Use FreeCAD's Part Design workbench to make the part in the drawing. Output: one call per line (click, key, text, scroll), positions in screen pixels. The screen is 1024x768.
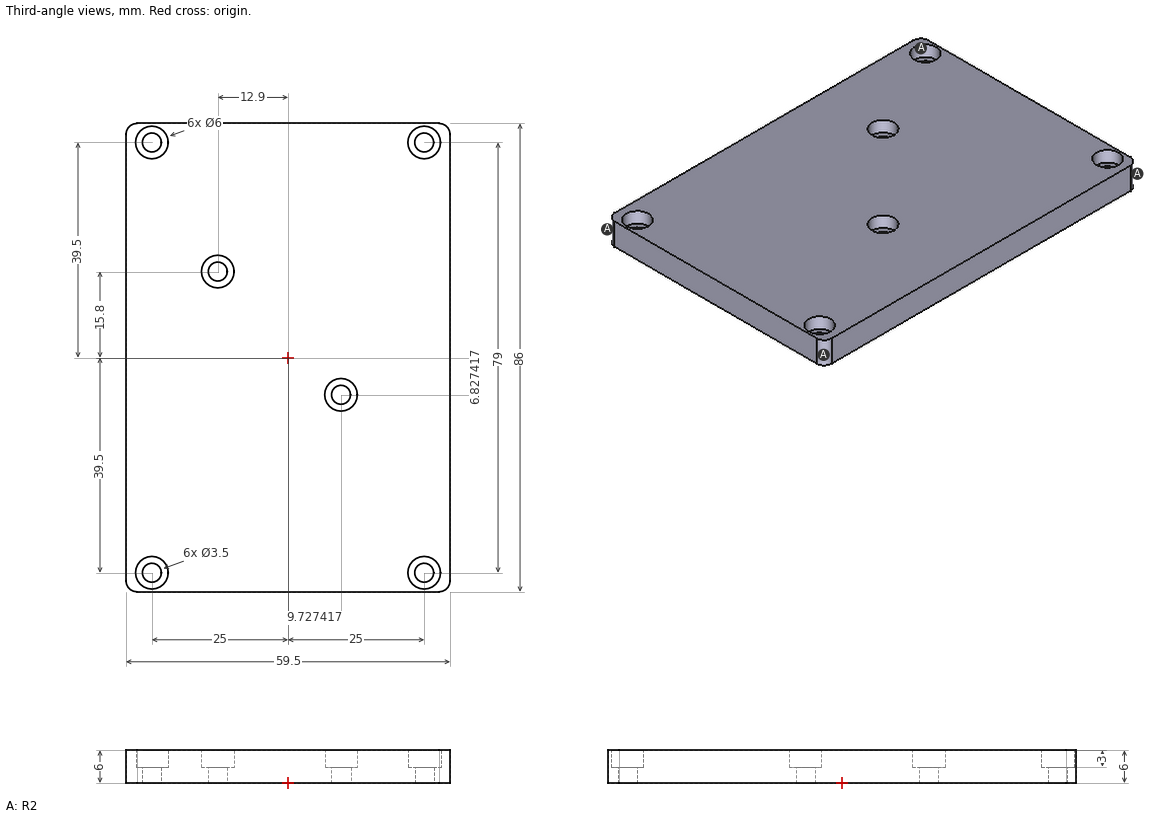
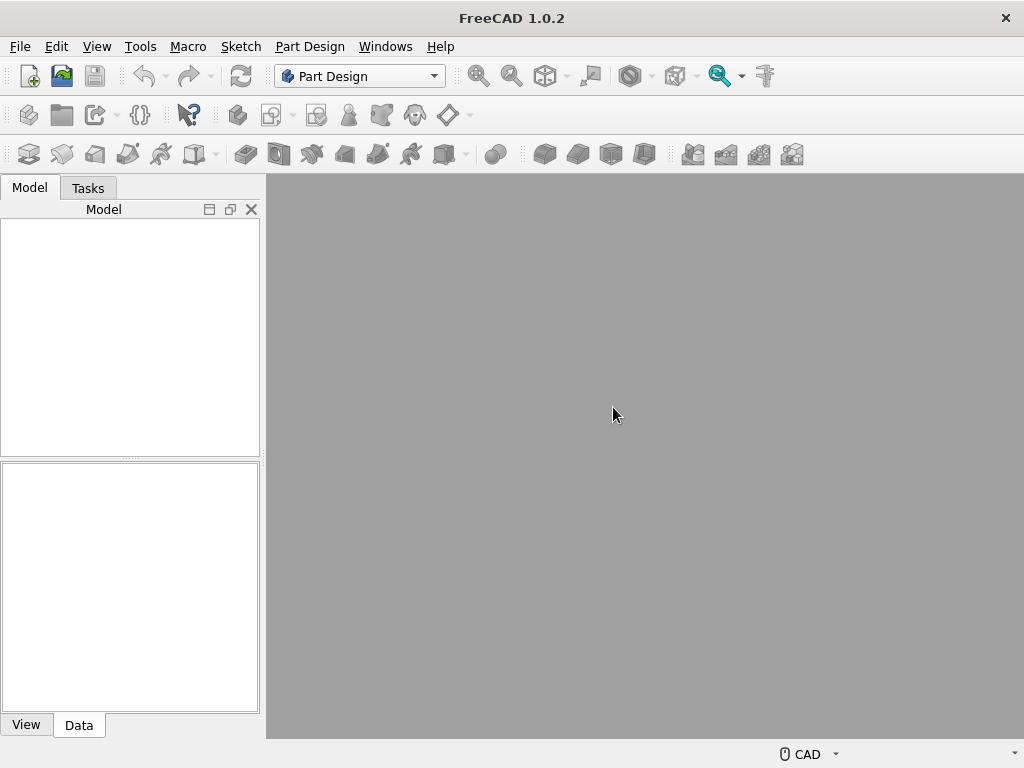
click(29, 76)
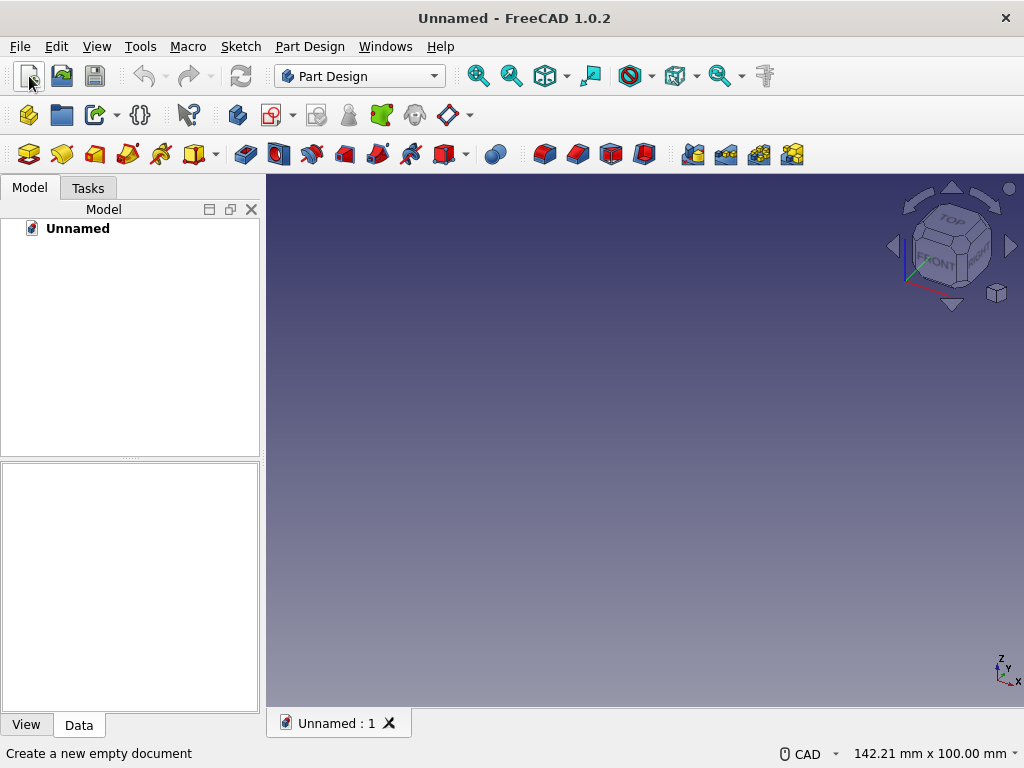
click(270, 116)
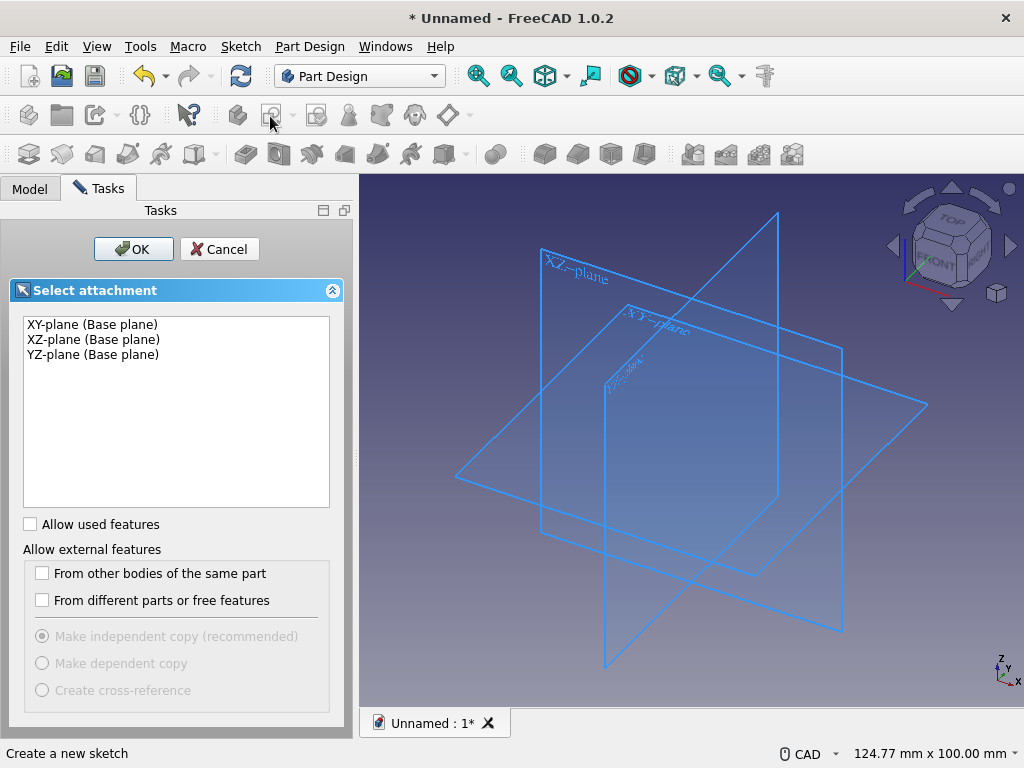
click(84, 324)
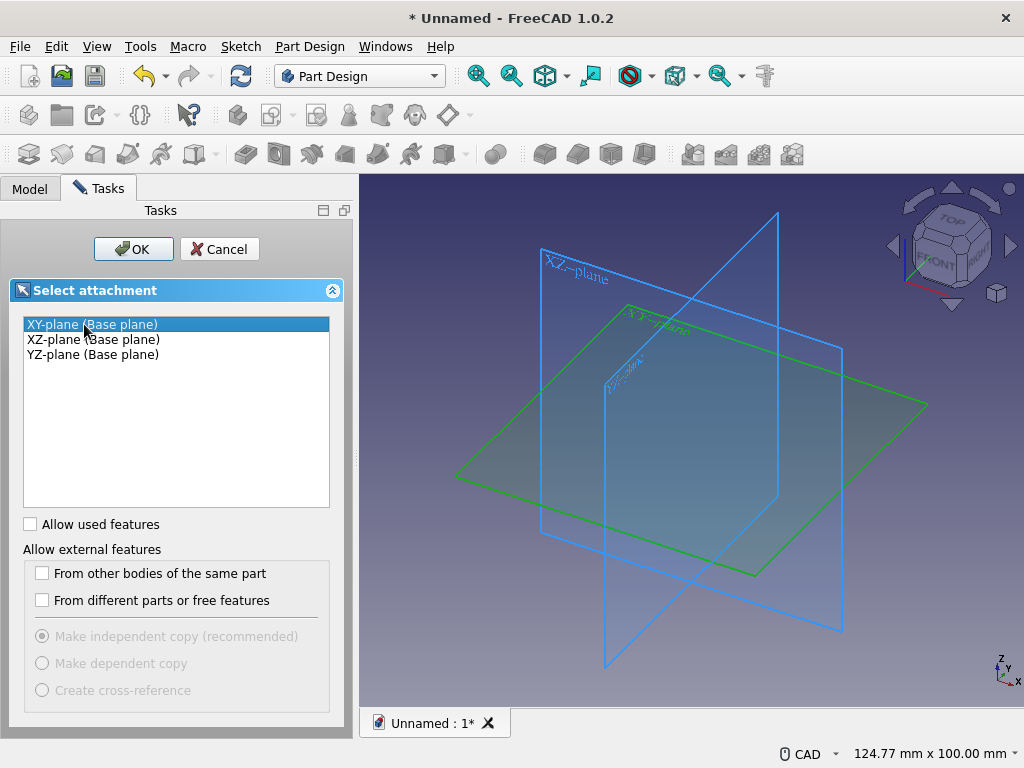
click(134, 249)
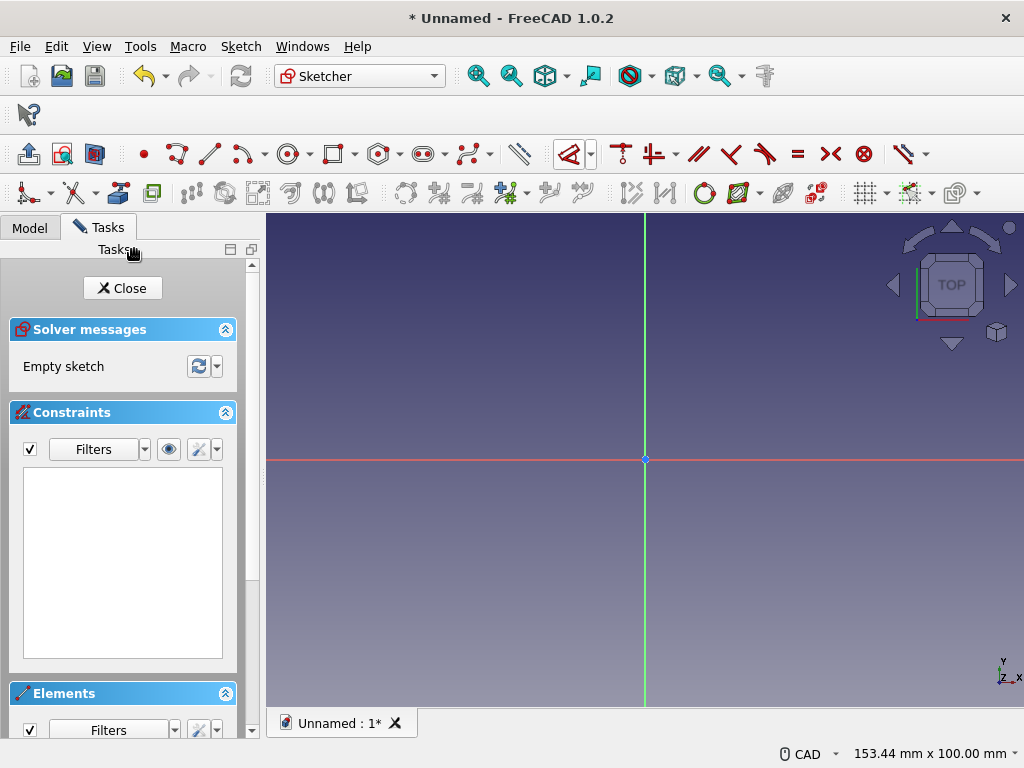
scroll(437, 460, down, 2)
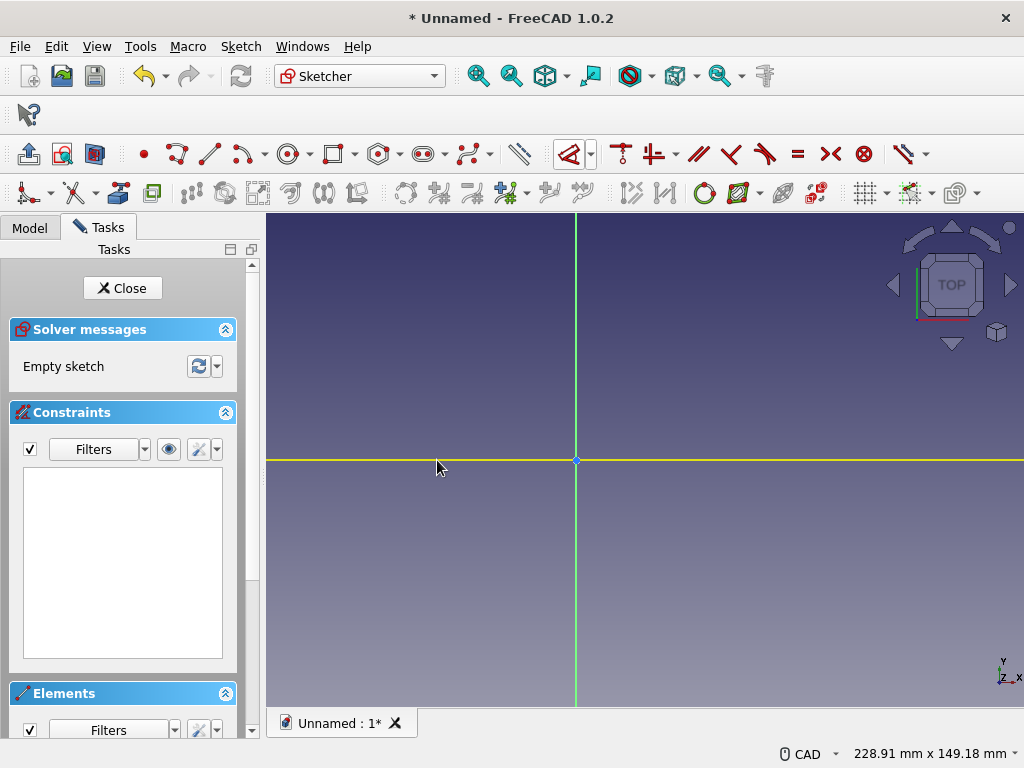
click(354, 154)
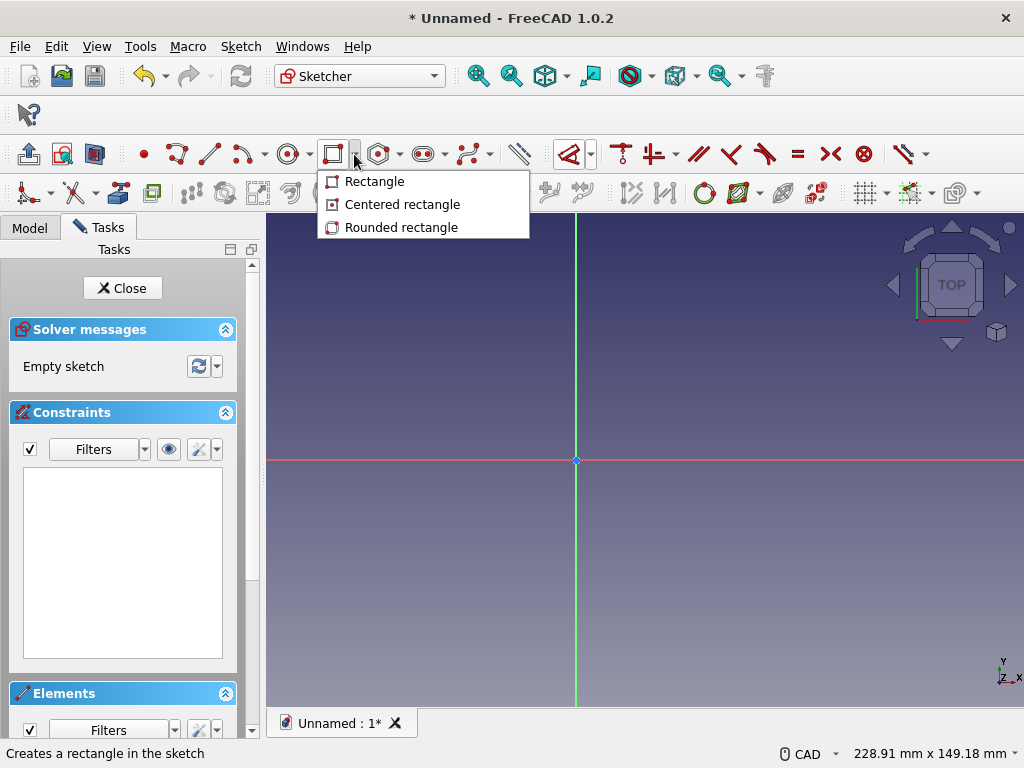
click(424, 204)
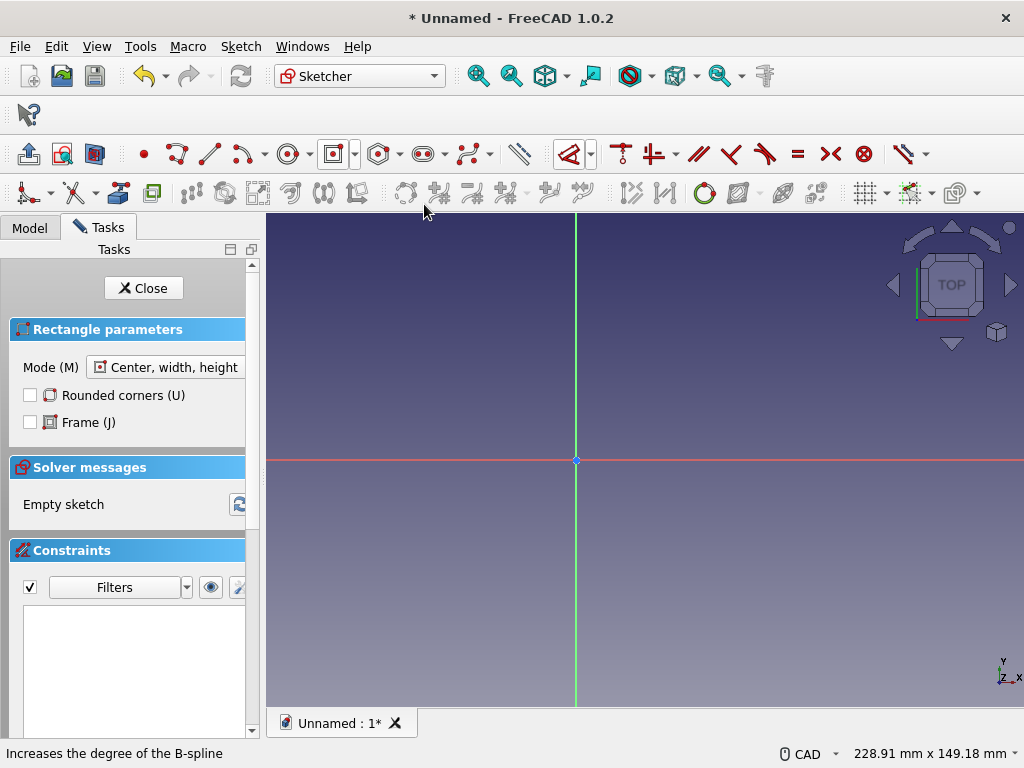
click(577, 460)
click(675, 318)
key(Escape)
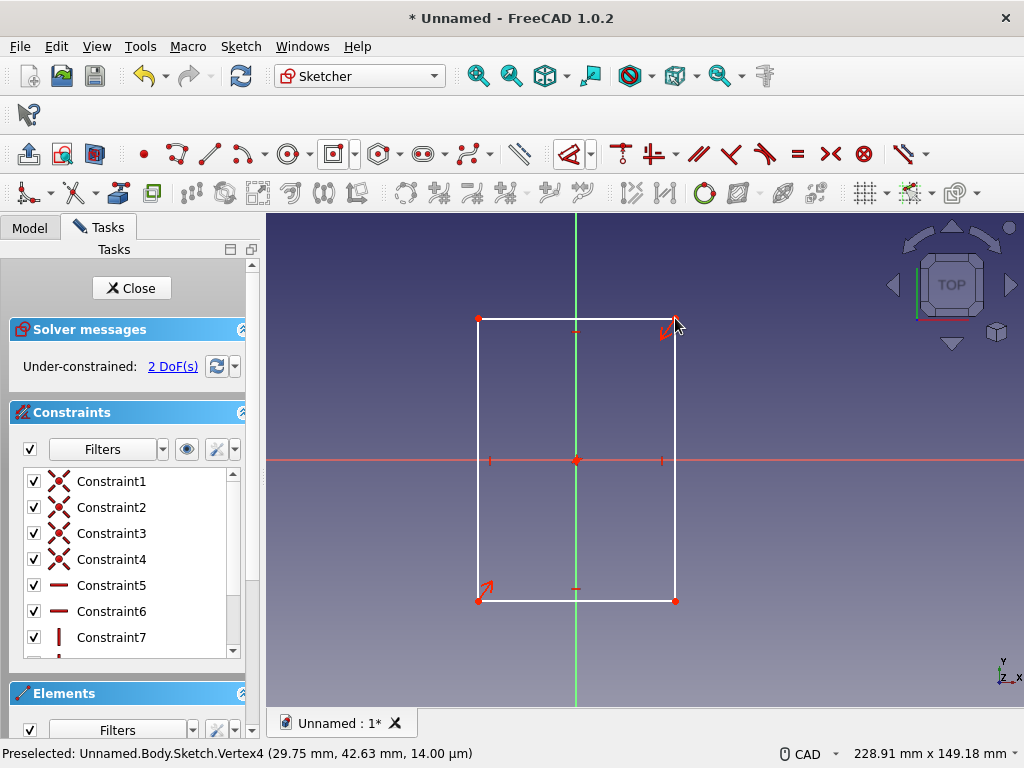
key(d)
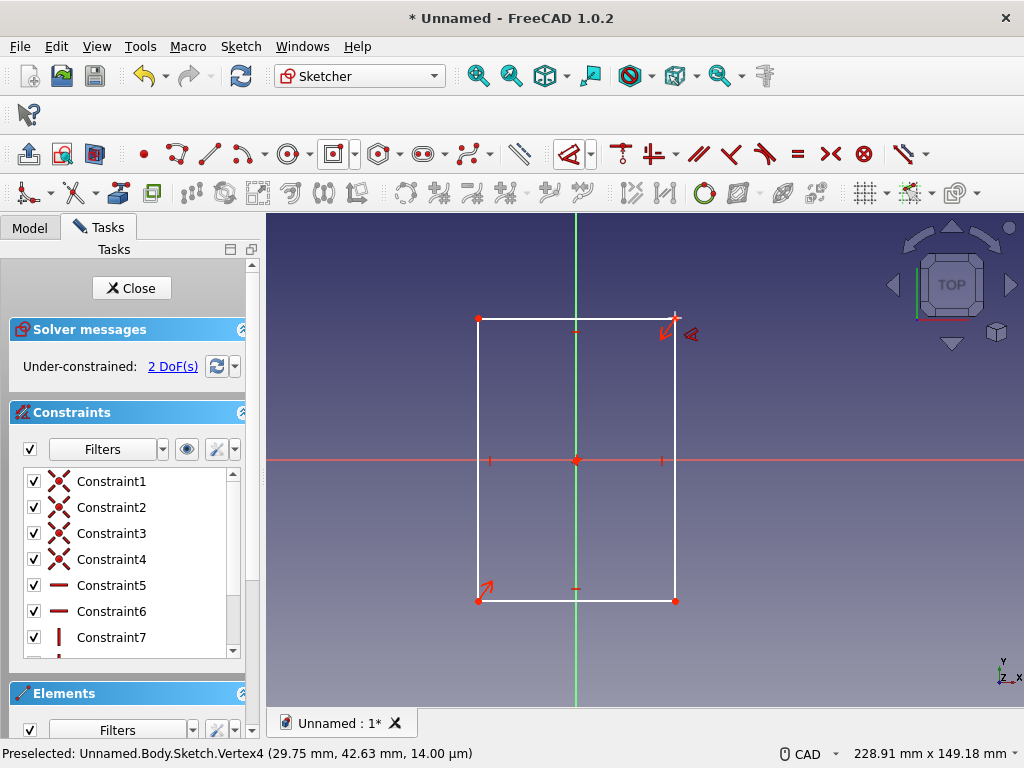
click(675, 517)
click(709, 395)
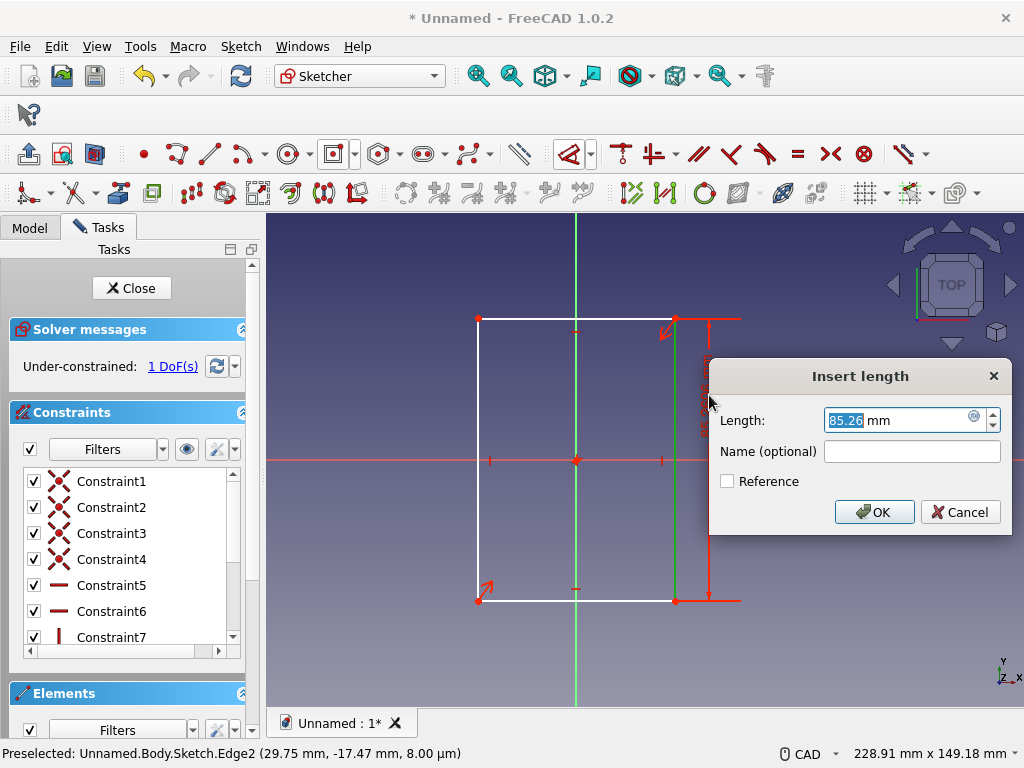
text(86)
key(Return)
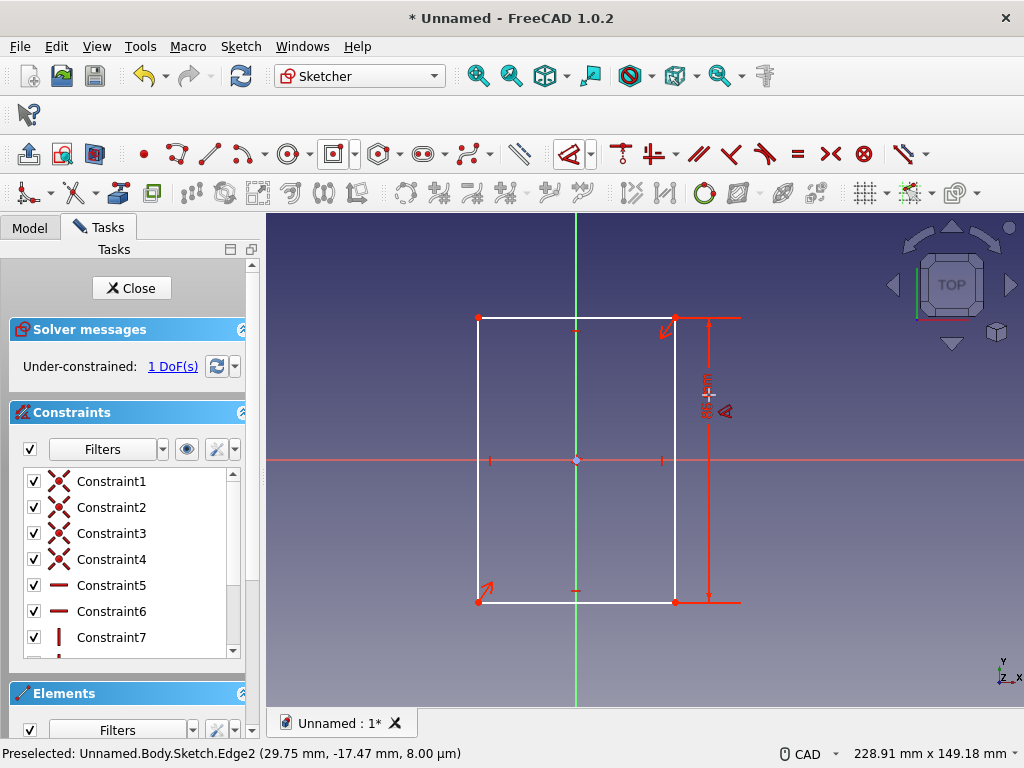
click(537, 603)
click(531, 637)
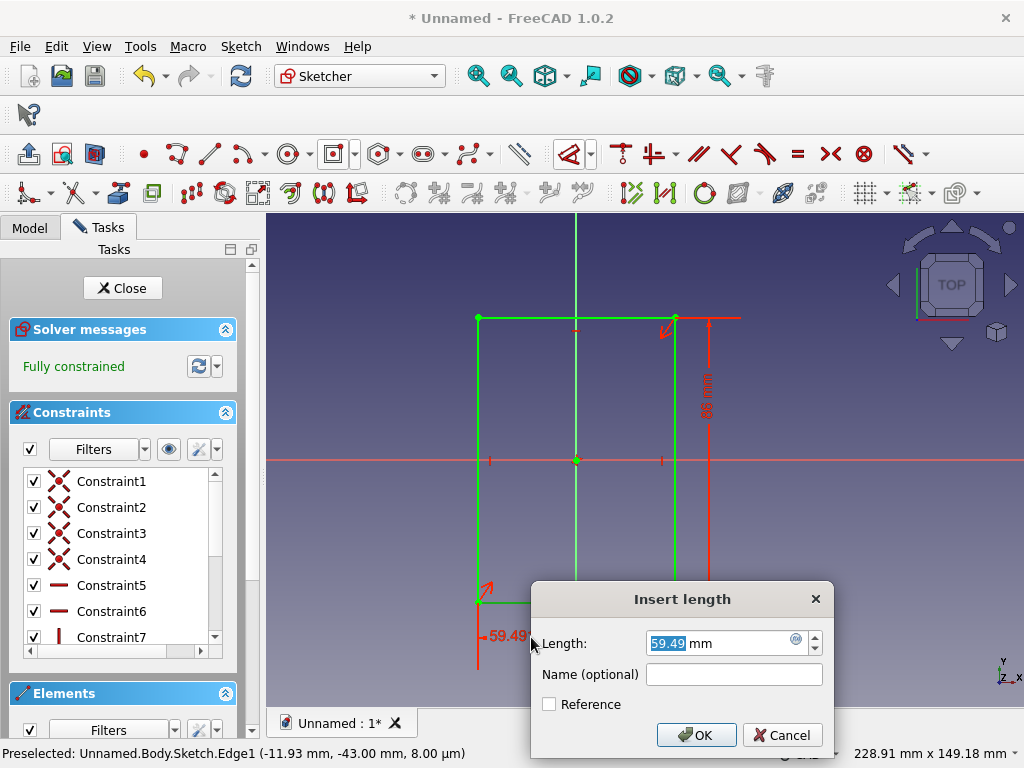
text(59.5)
key(Return)
key(Escape)